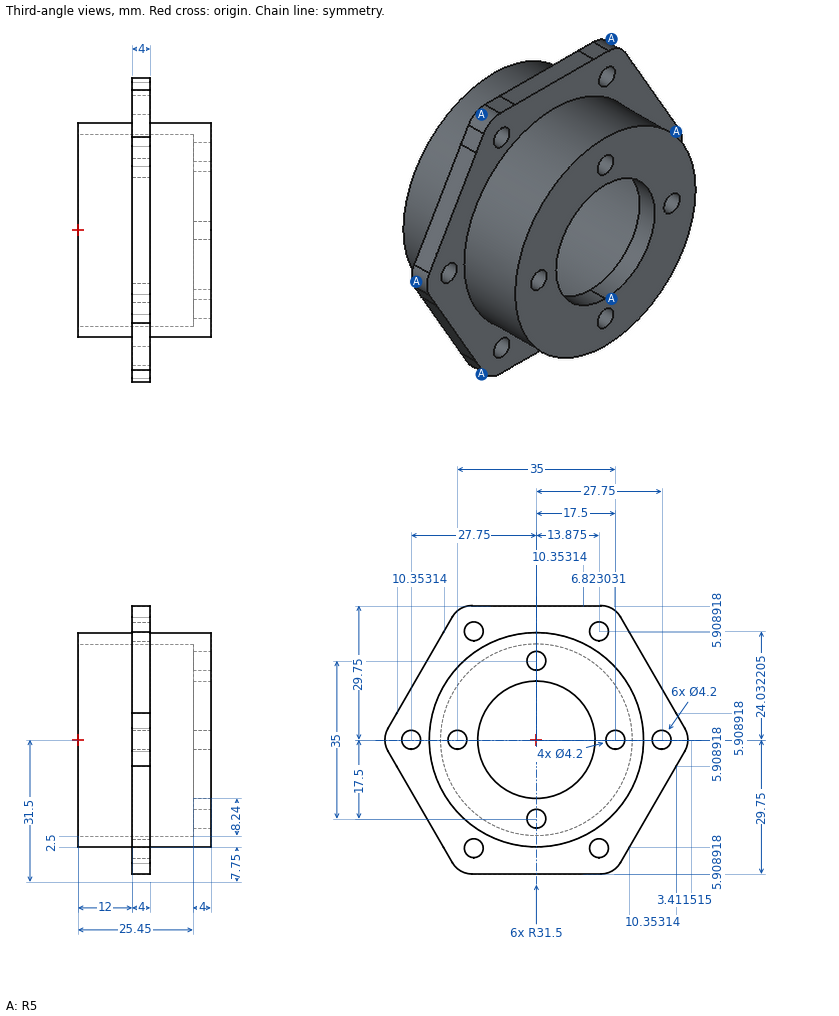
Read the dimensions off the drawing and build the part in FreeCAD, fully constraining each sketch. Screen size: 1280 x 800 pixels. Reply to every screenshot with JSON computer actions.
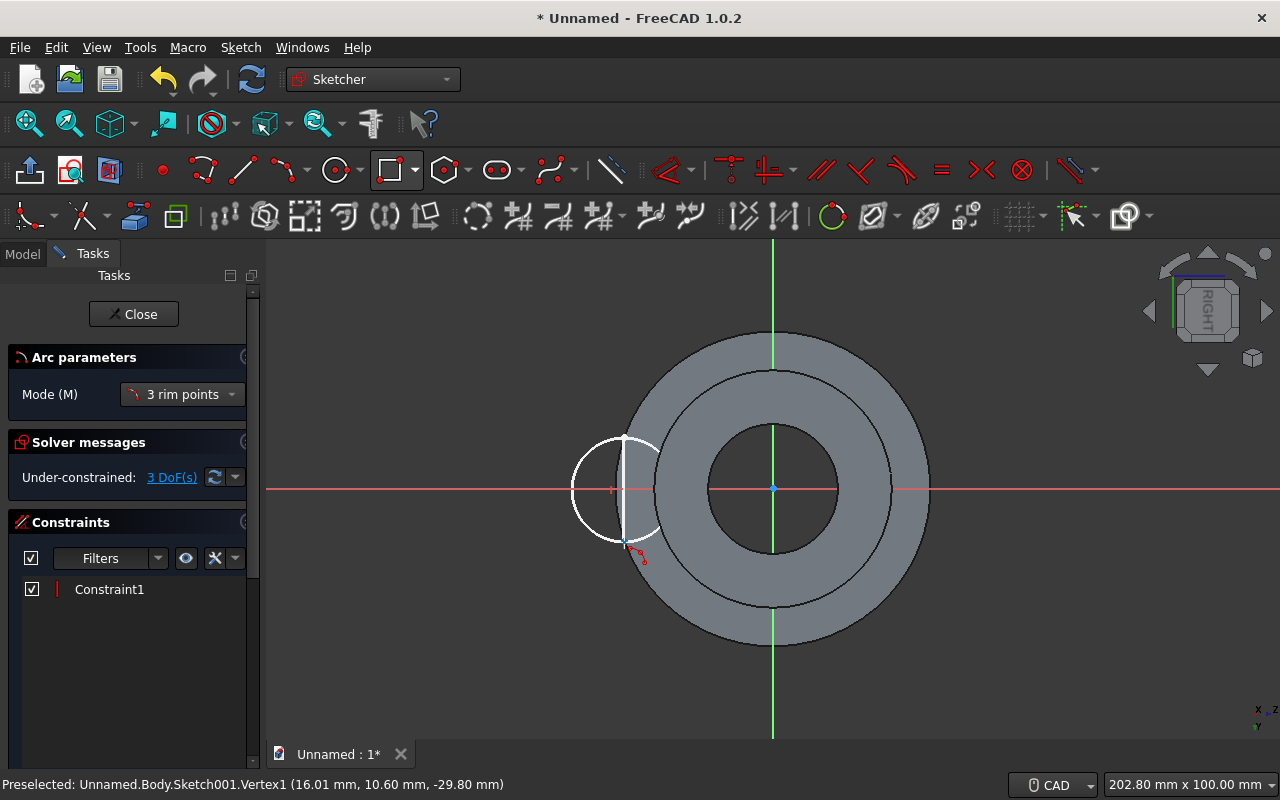
{"action": "scroll", "coordinate": [616, 500], "scroll_direction": "up", "scroll_amount": 4}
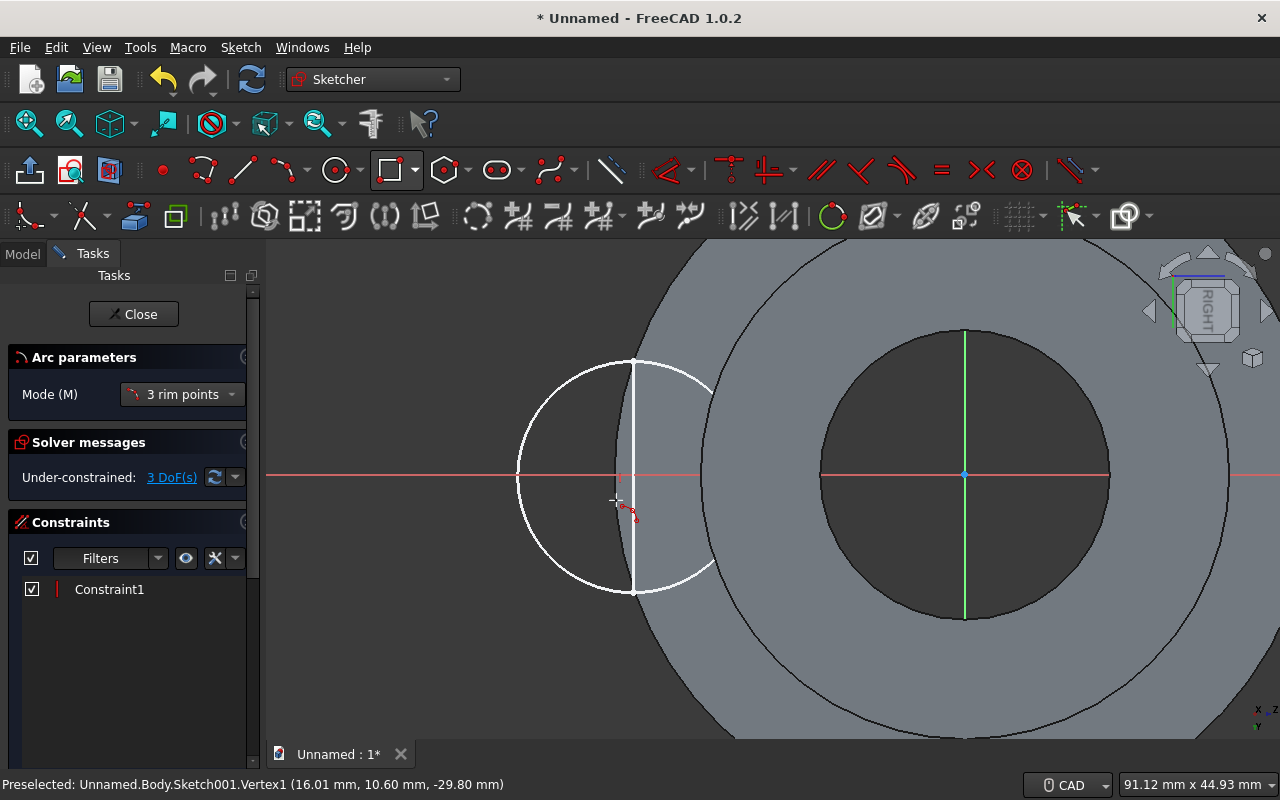
{"action": "left_click", "coordinate": [615, 498]}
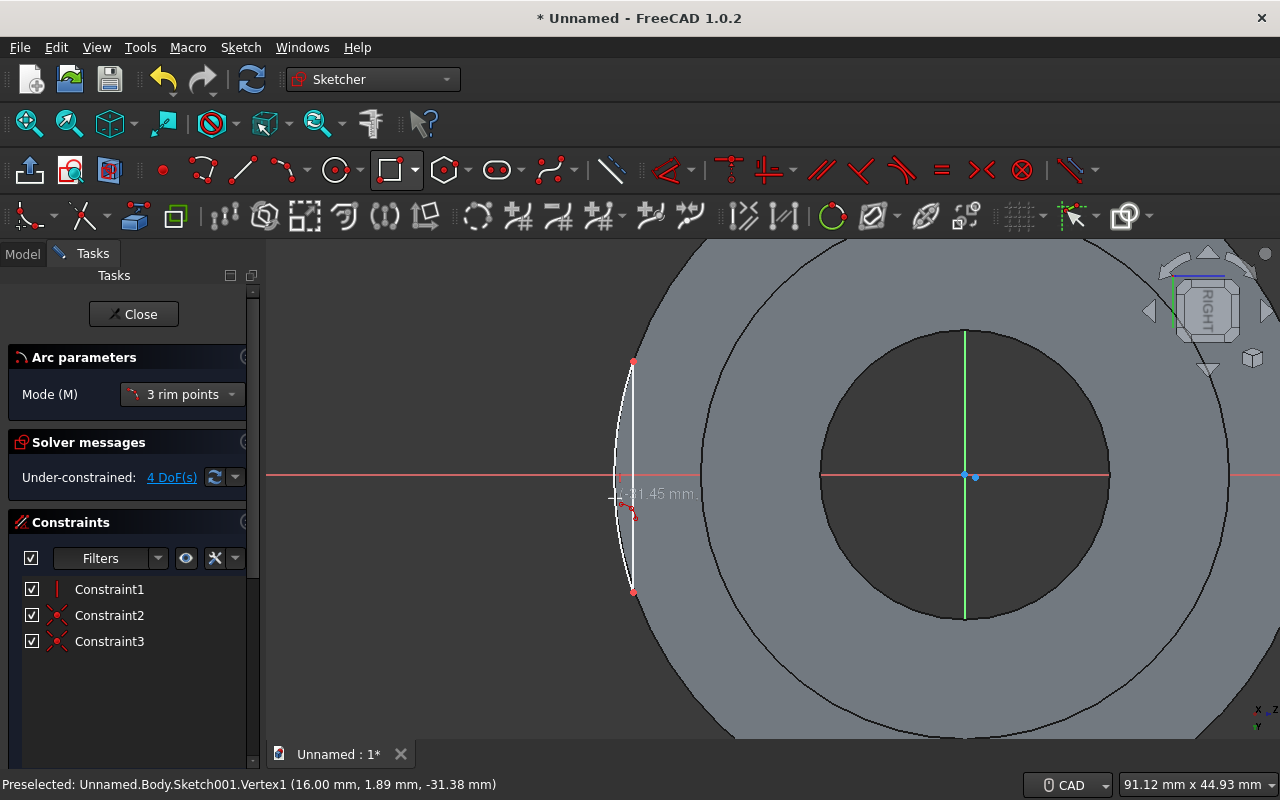
{"action": "key", "text": "g l"}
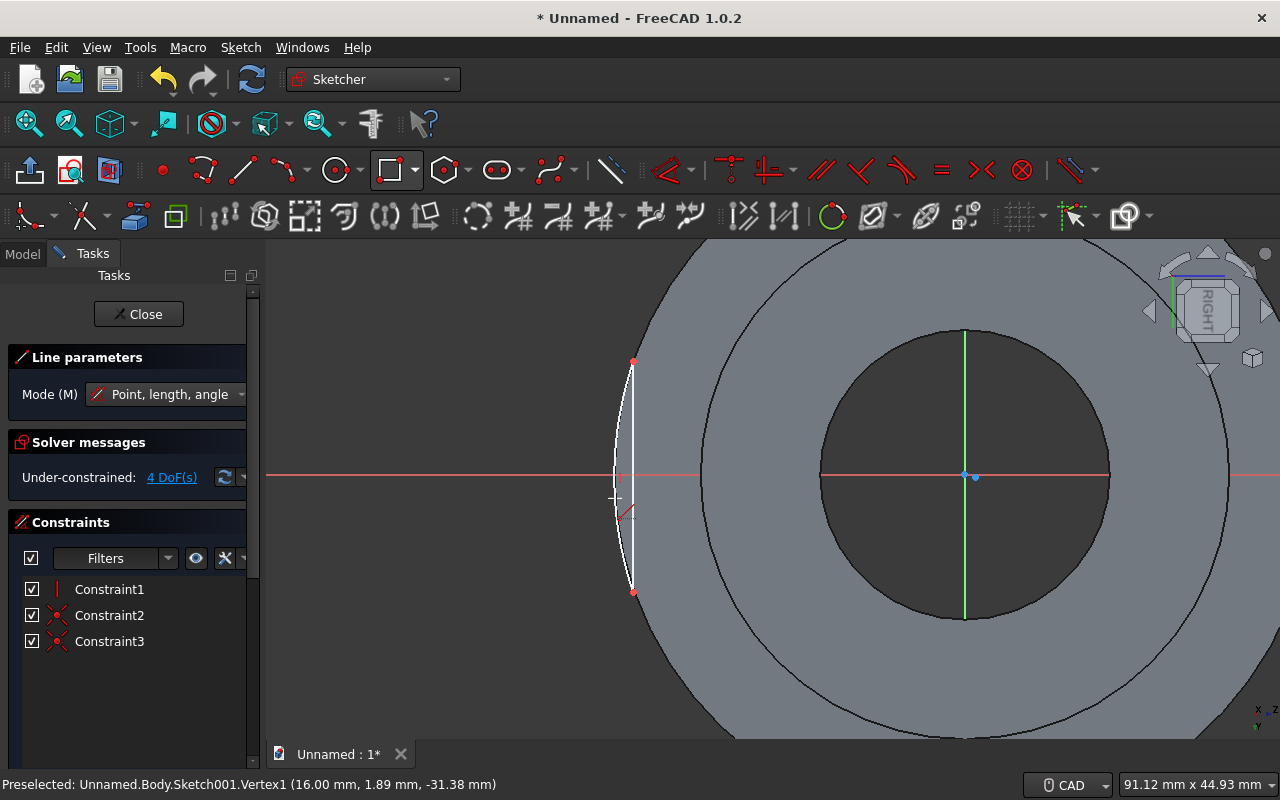
{"action": "scroll", "coordinate": [492, 501], "scroll_direction": "down", "scroll_amount": 4}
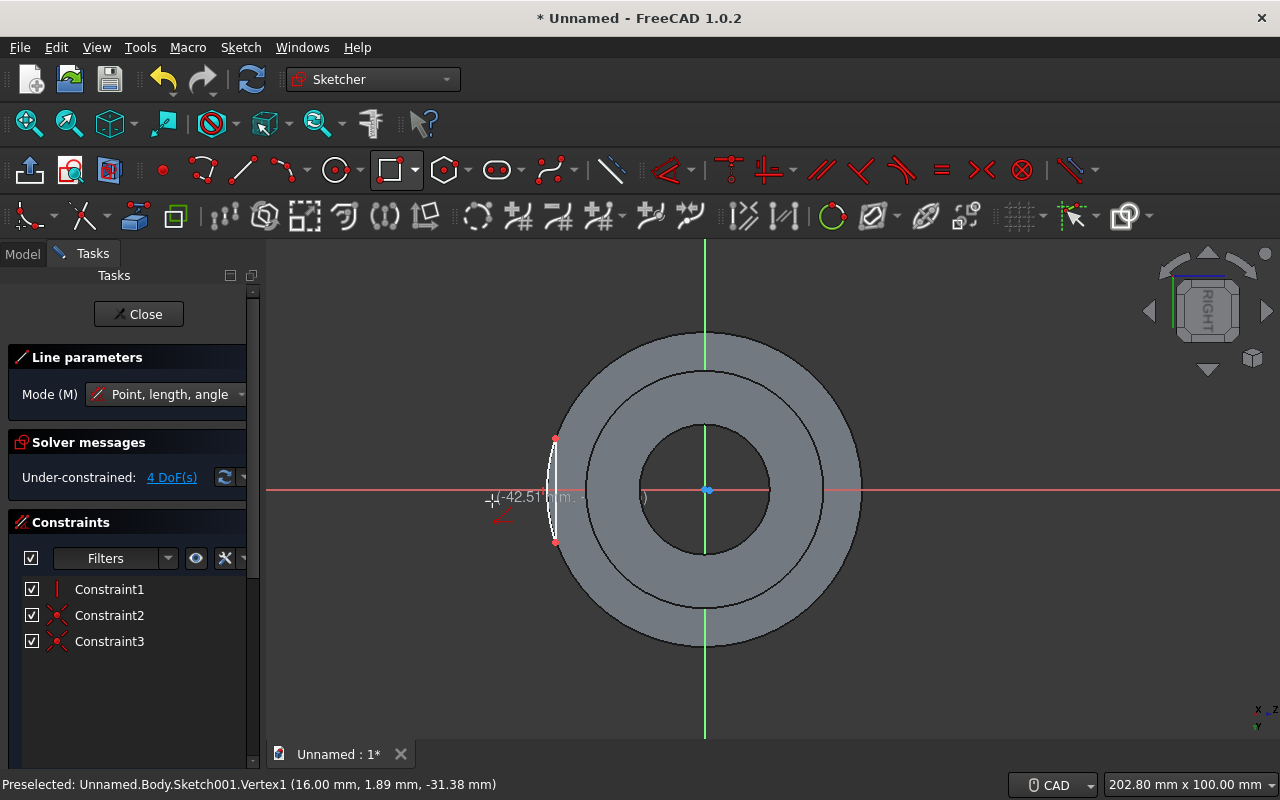
{"action": "left_click", "coordinate": [675, 644]}
{"action": "left_click", "coordinate": [585, 592]}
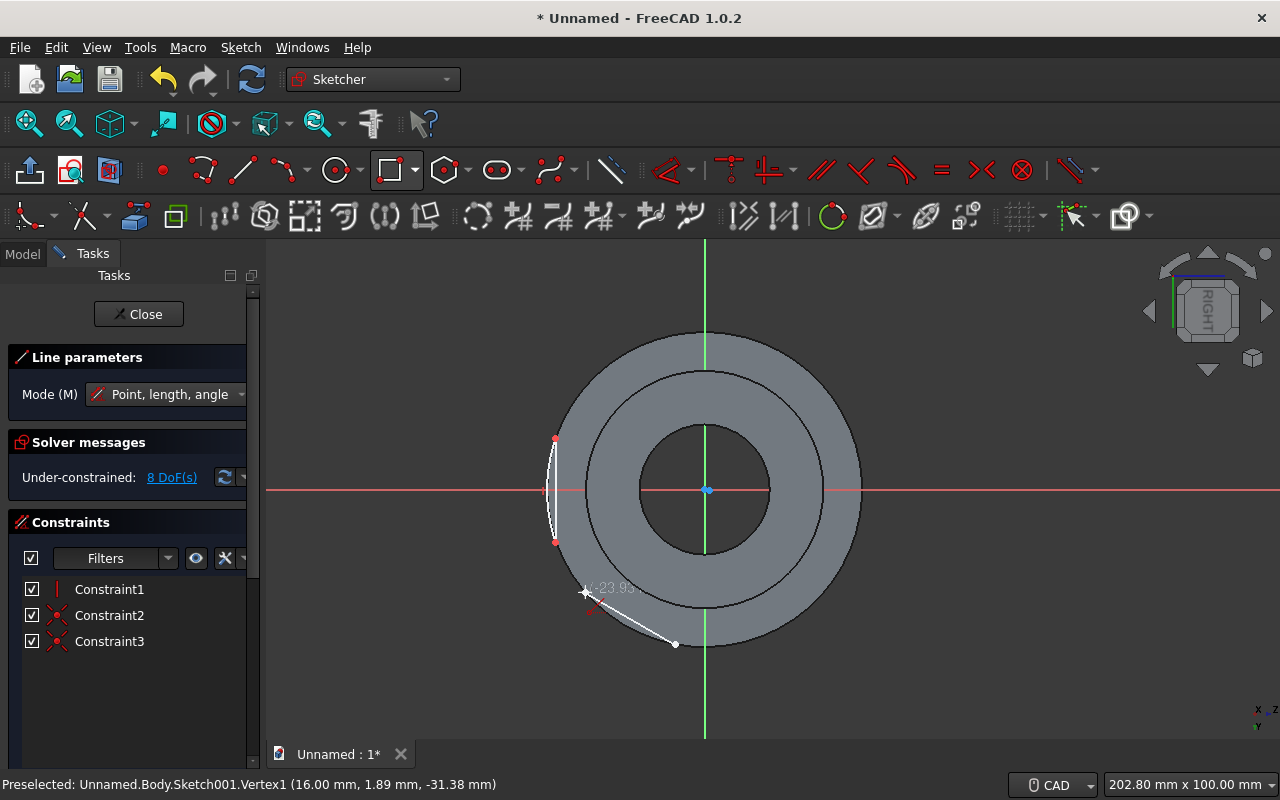
{"action": "key", "text": "g 3 a"}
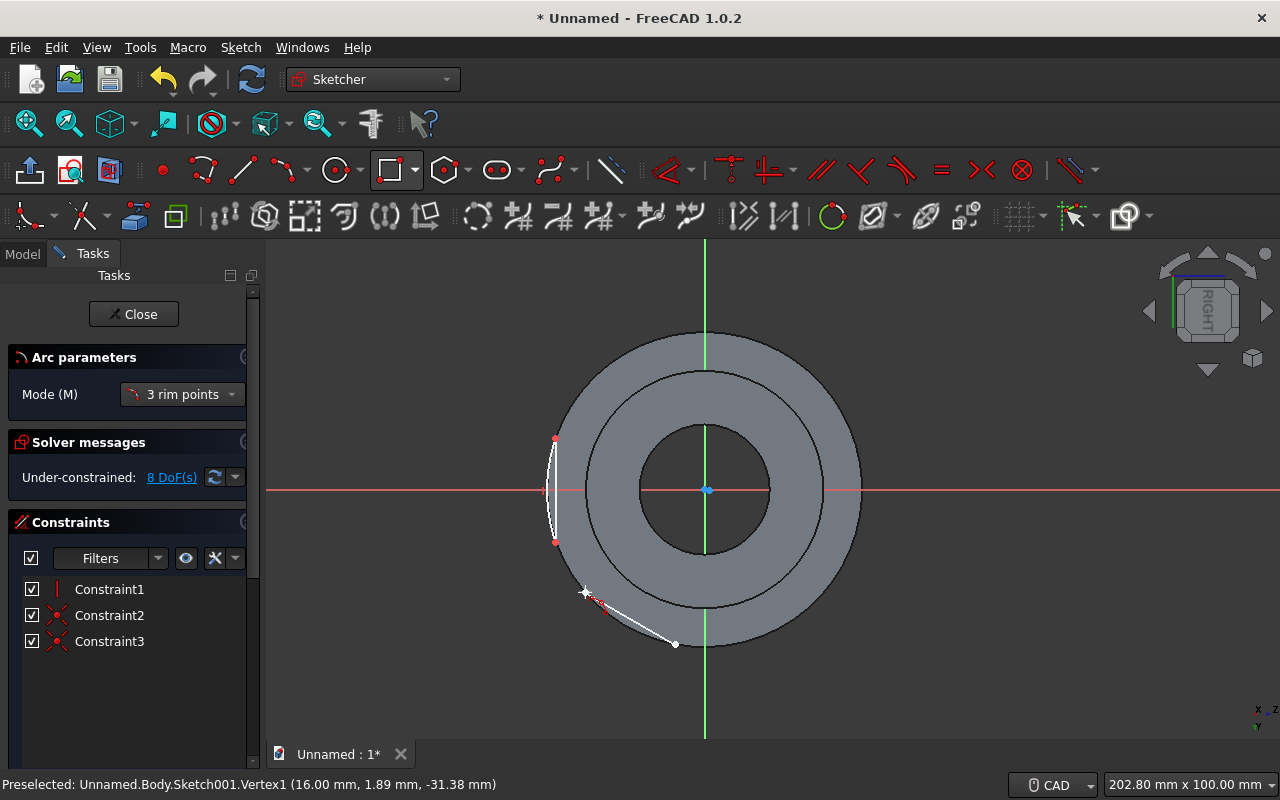
{"action": "left_click", "coordinate": [585, 593]}
{"action": "left_click", "coordinate": [675, 645]}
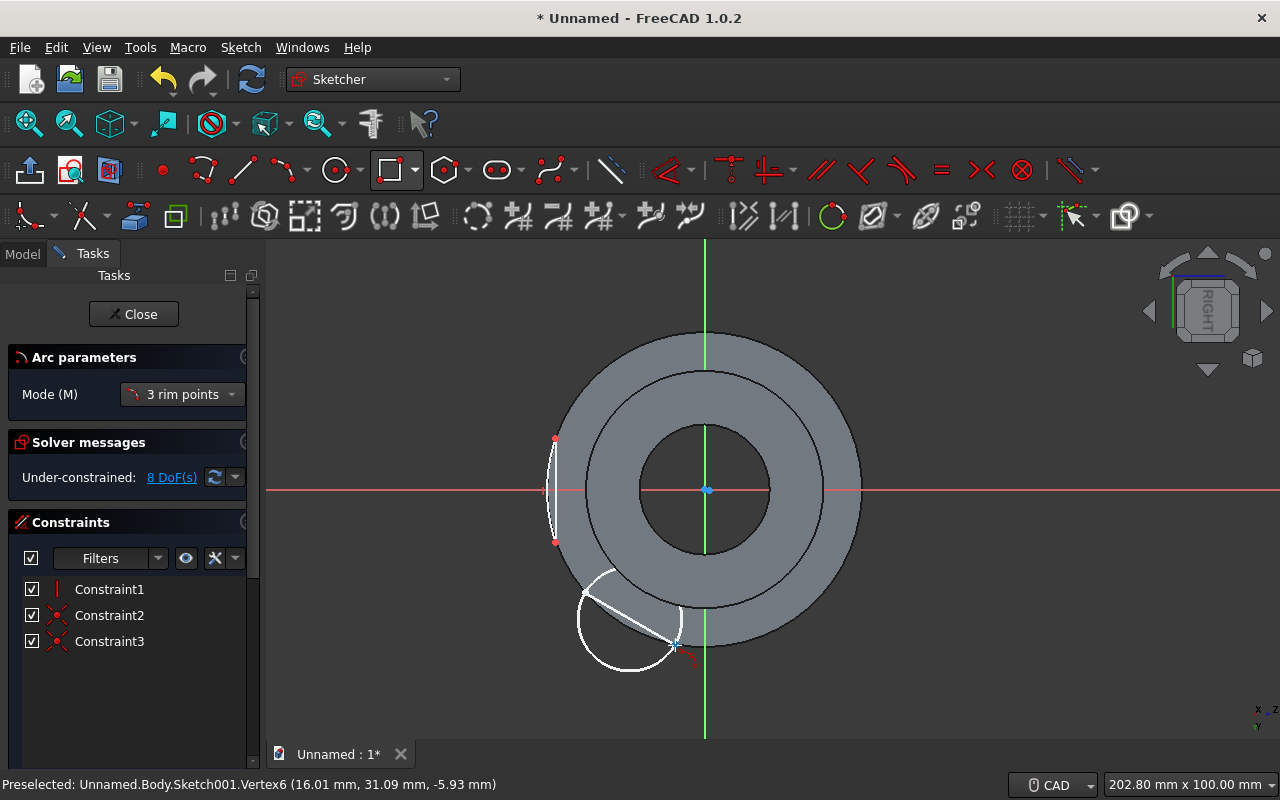
{"action": "scroll", "coordinate": [626, 626], "scroll_direction": "up", "scroll_amount": 3}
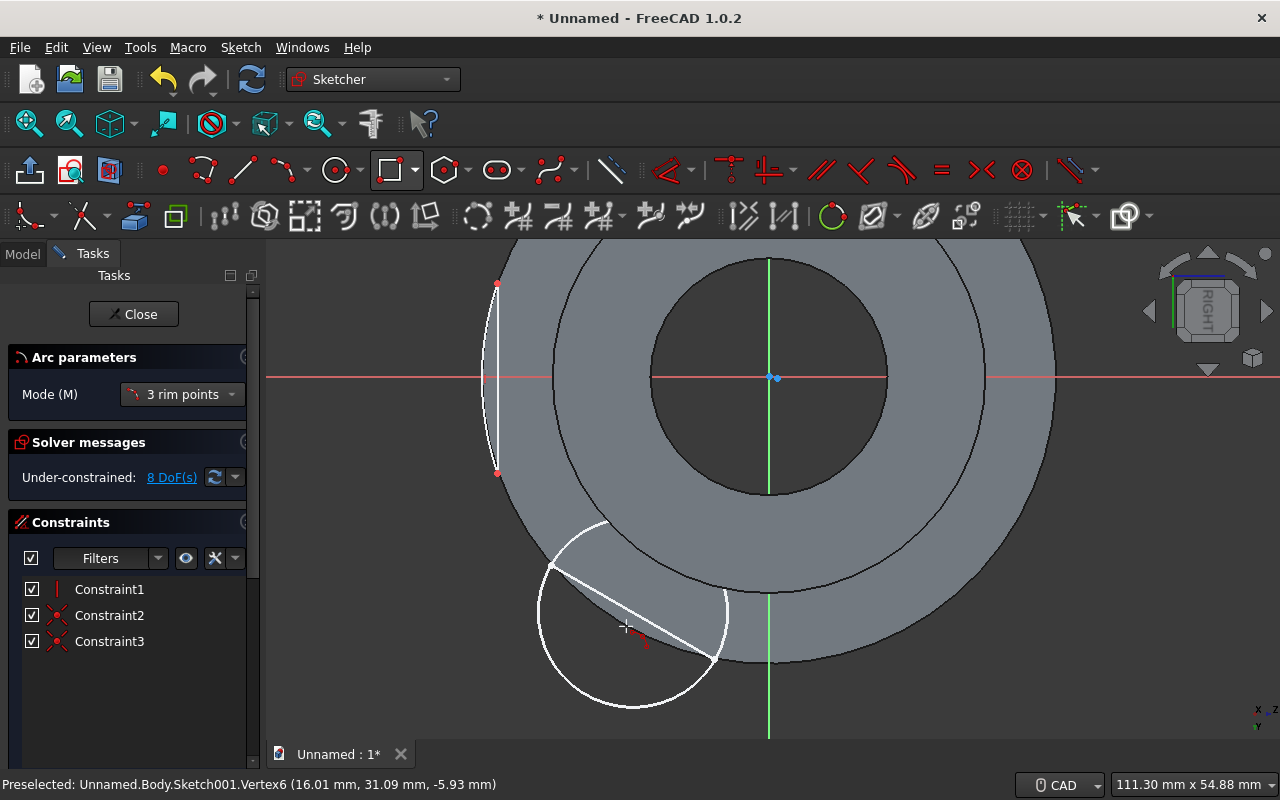
{"action": "left_click", "coordinate": [626, 625]}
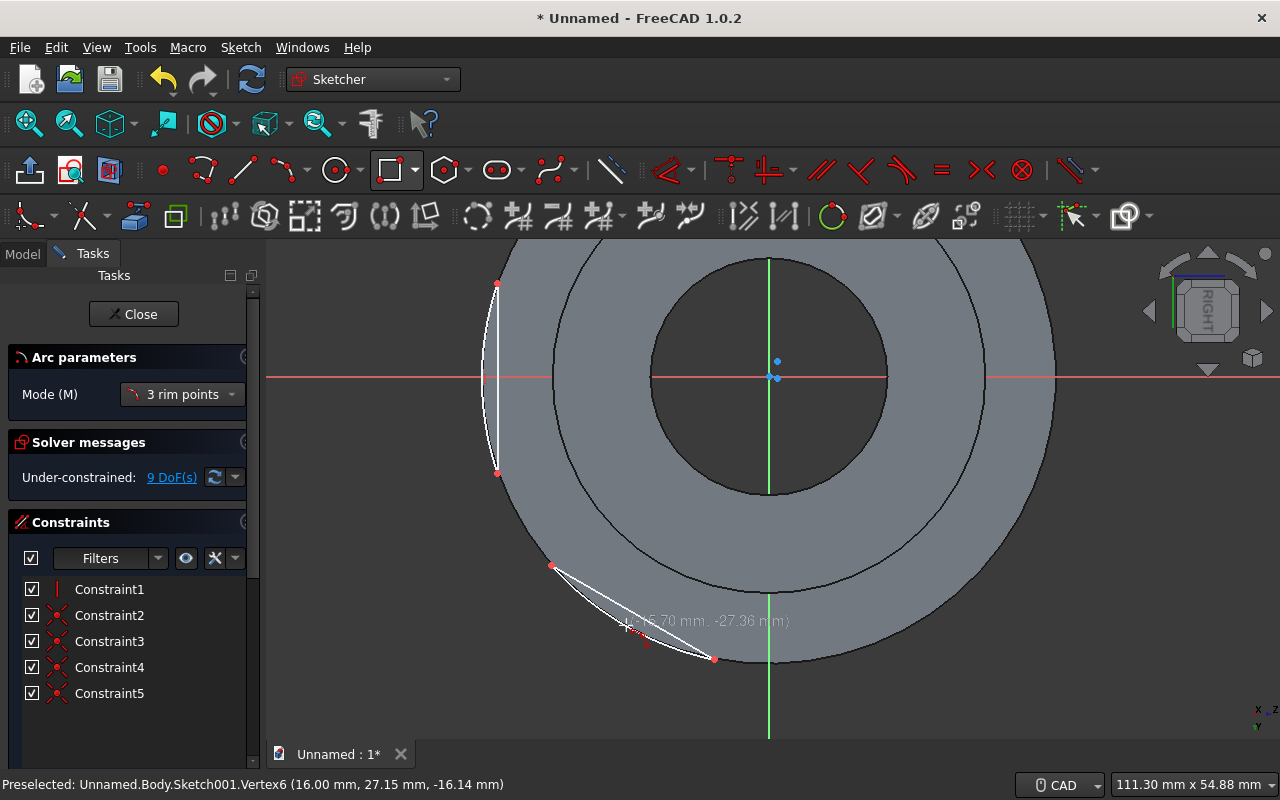
{"action": "key", "text": "g l"}